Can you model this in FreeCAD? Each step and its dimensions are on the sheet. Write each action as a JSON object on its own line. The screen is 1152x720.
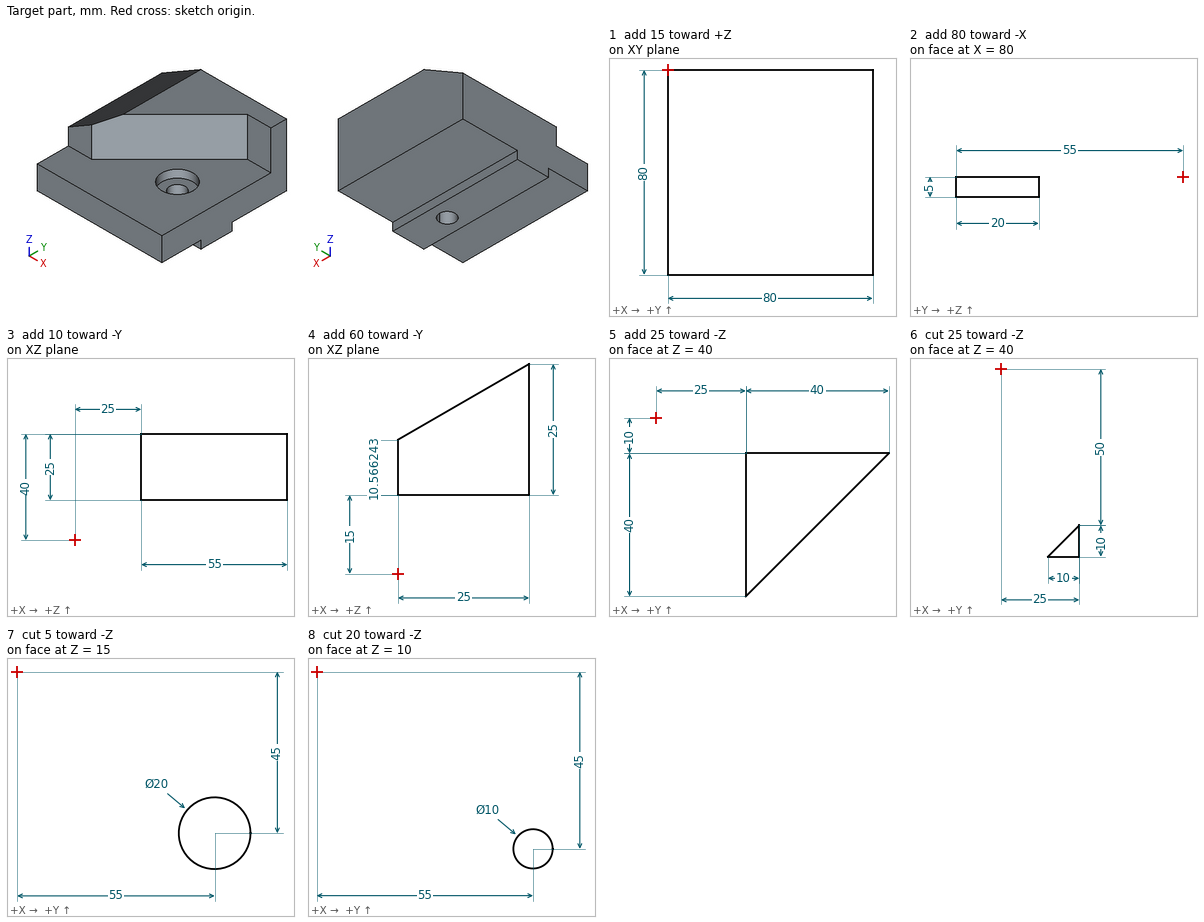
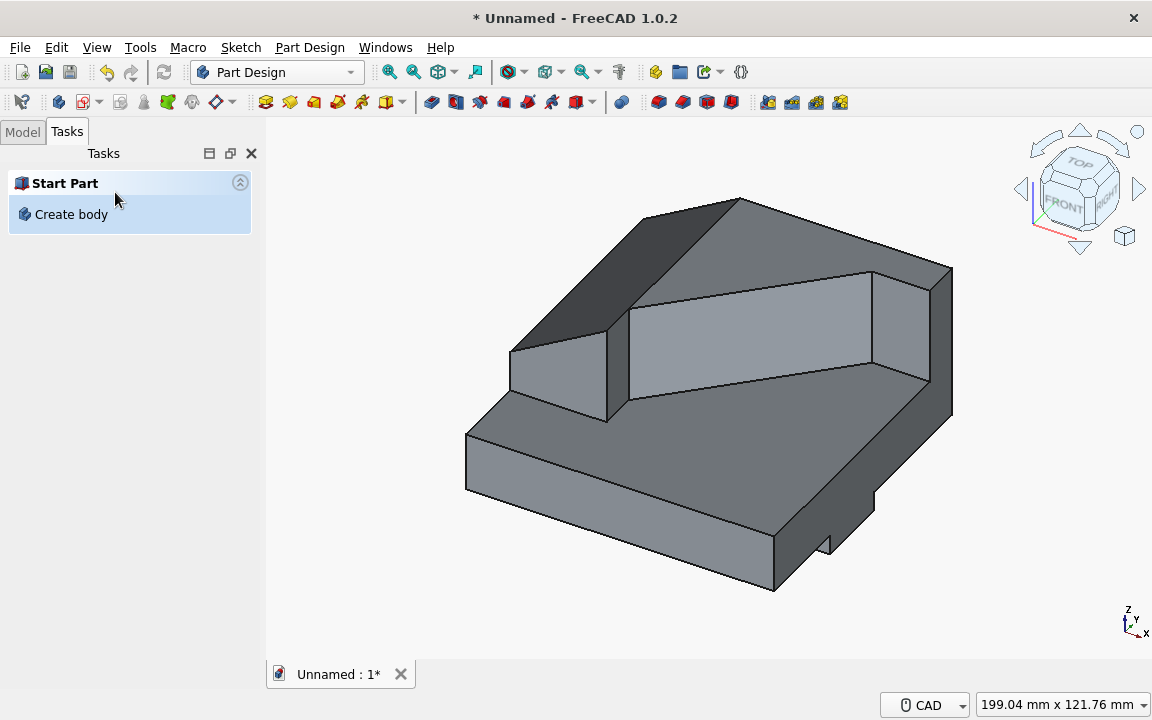
{"action": "left_click", "coordinate": [746, 252]}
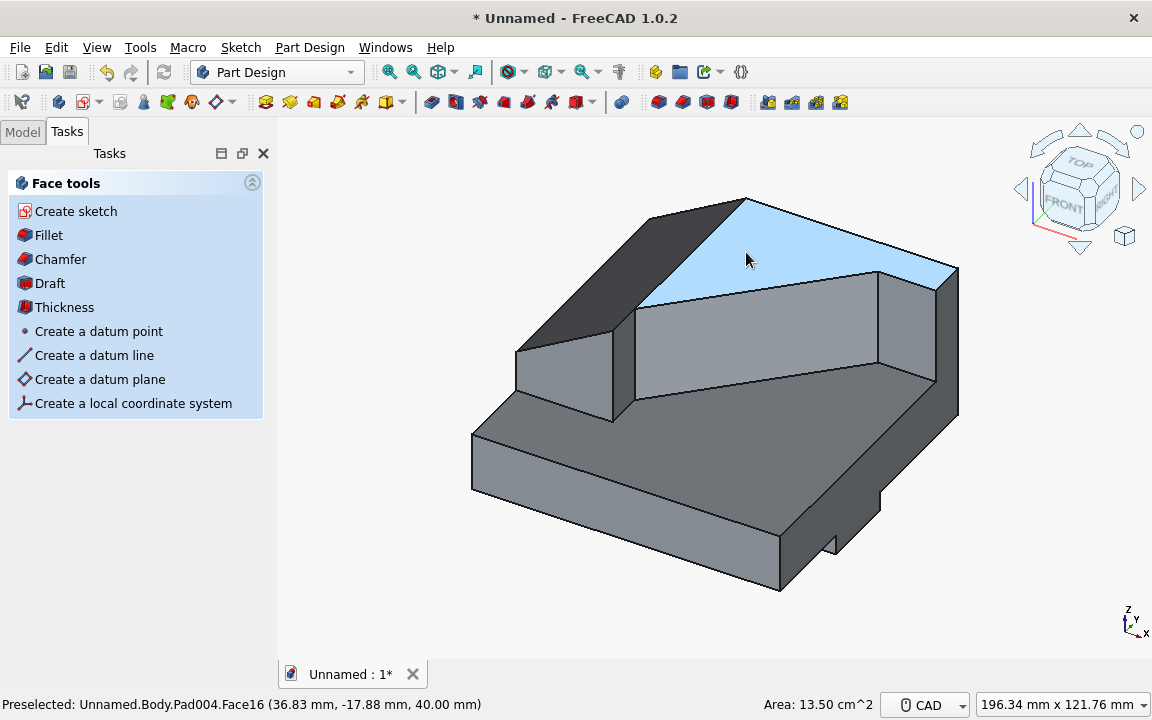
{"action": "left_click", "coordinate": [84, 102]}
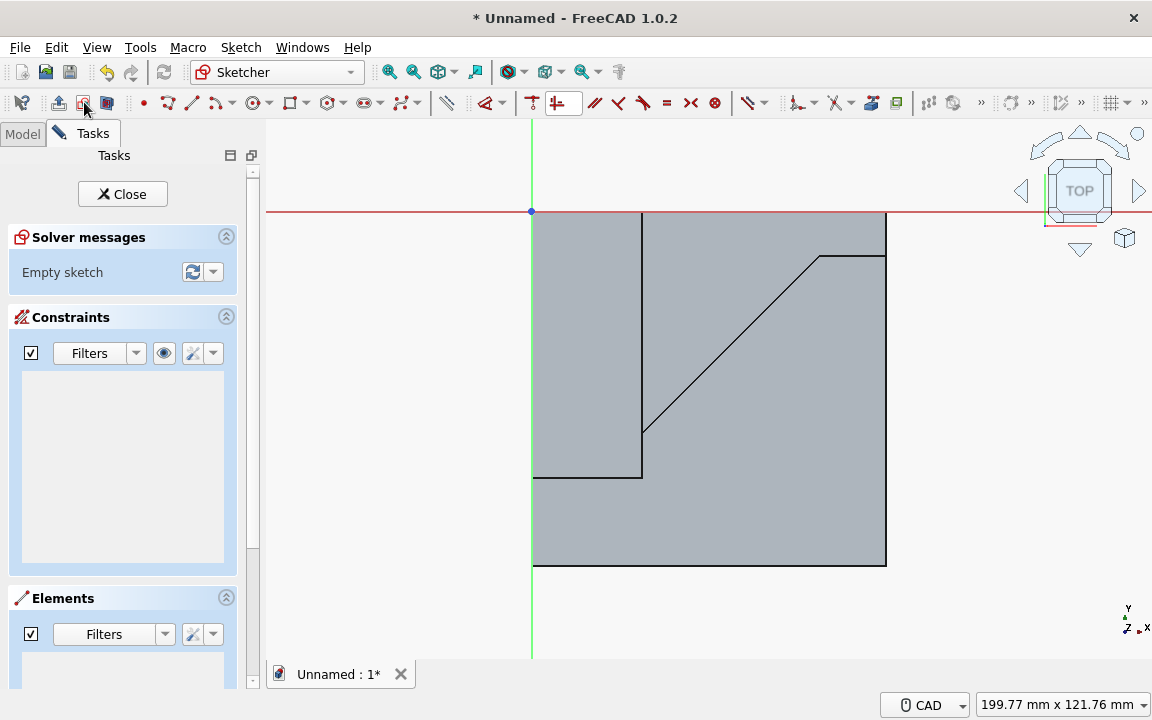
{"action": "scroll", "coordinate": [617, 466], "scroll_direction": "up", "scroll_amount": 10}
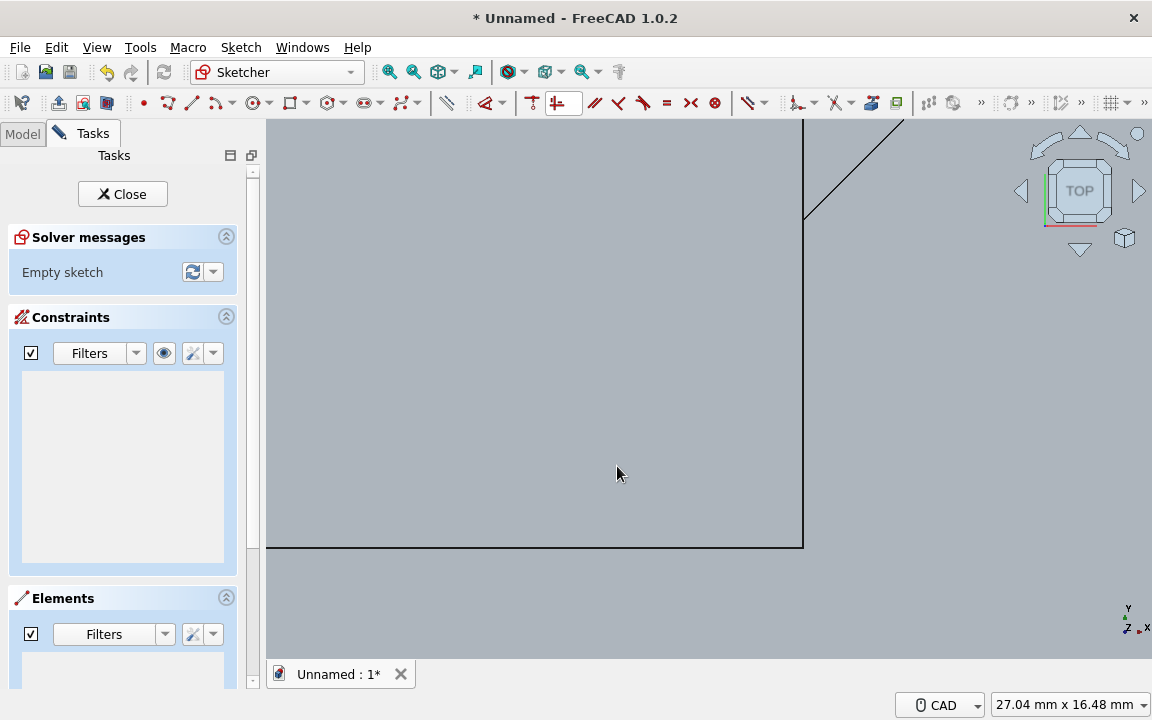
{"action": "left_click", "coordinate": [168, 104]}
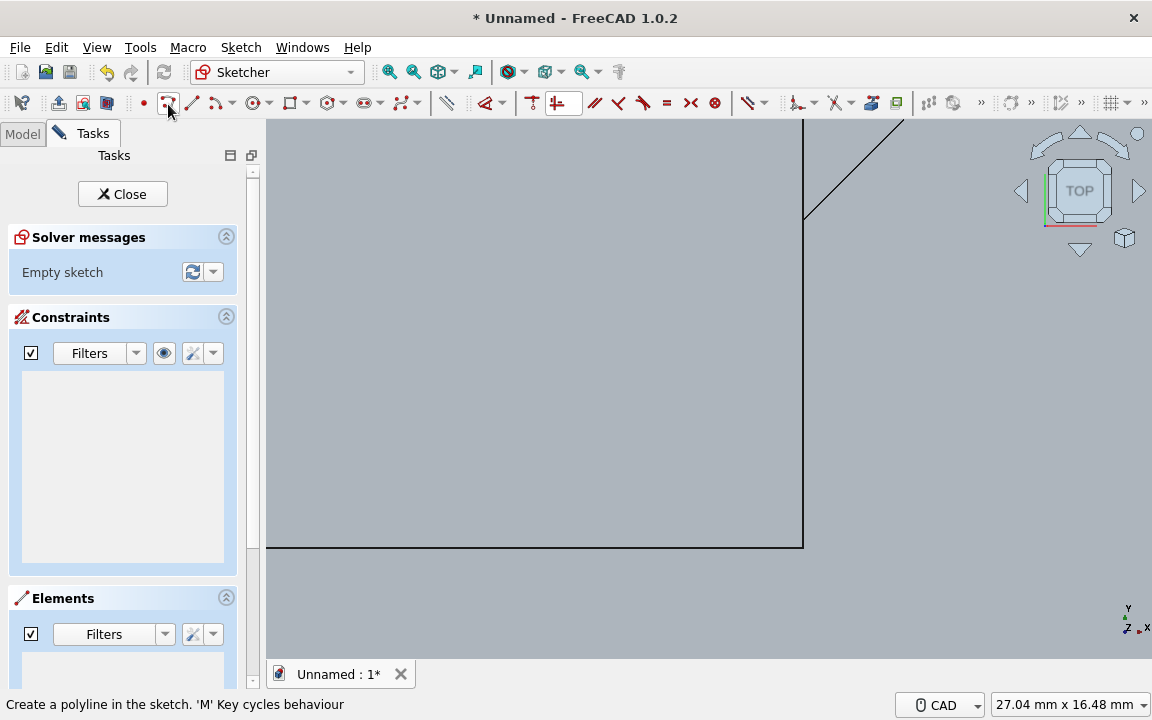
{"action": "left_click", "coordinate": [803, 221]}
{"action": "left_click", "coordinate": [475, 548]}
{"action": "left_click", "coordinate": [803, 548]}
{"action": "left_click", "coordinate": [803, 222]}
{"action": "key", "text": "Escape"}
{"action": "key", "text": "Escape"}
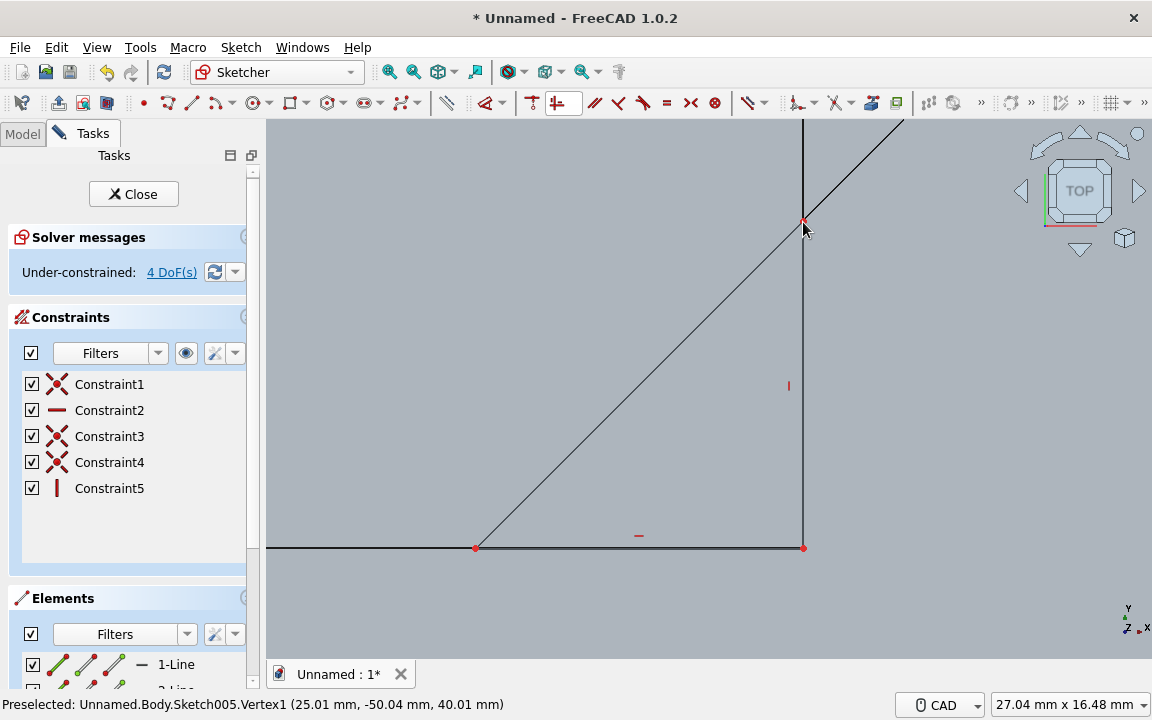
{"action": "left_click", "coordinate": [486, 104]}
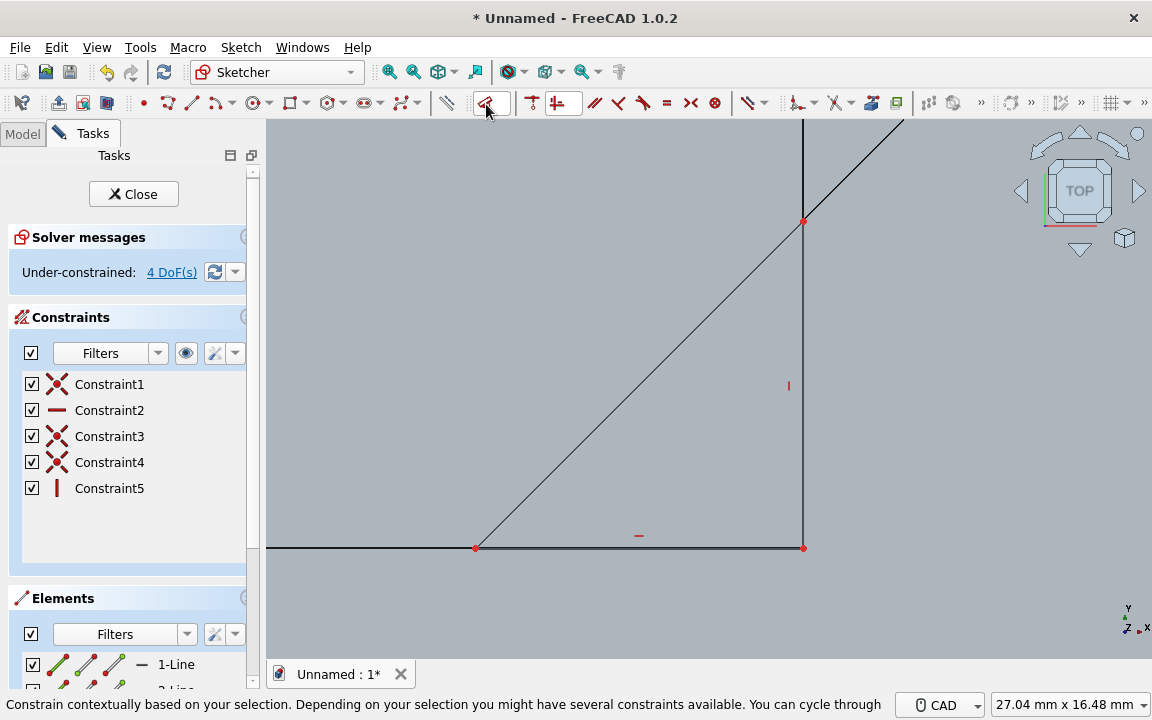
{"action": "left_click", "coordinate": [573, 549]}
{"action": "left_click", "coordinate": [639, 583]}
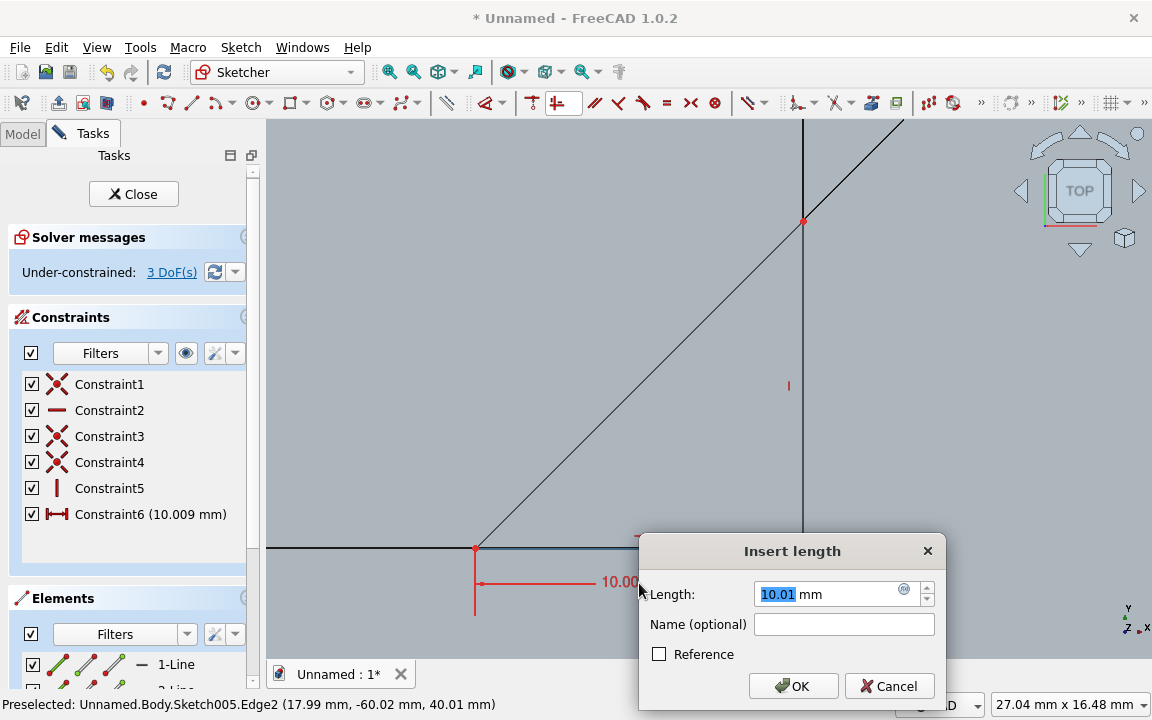
{"action": "type", "text": "10"}
{"action": "key", "text": "Return"}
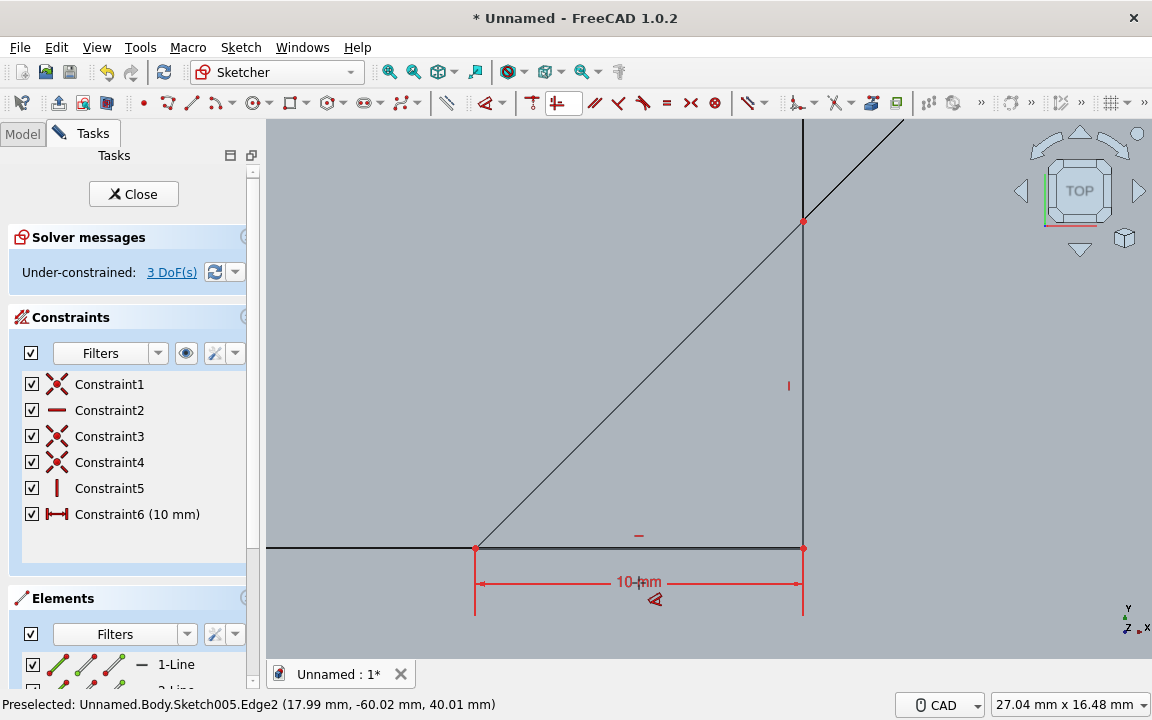
{"action": "left_click", "coordinate": [803, 451]}
{"action": "left_click", "coordinate": [837, 386]}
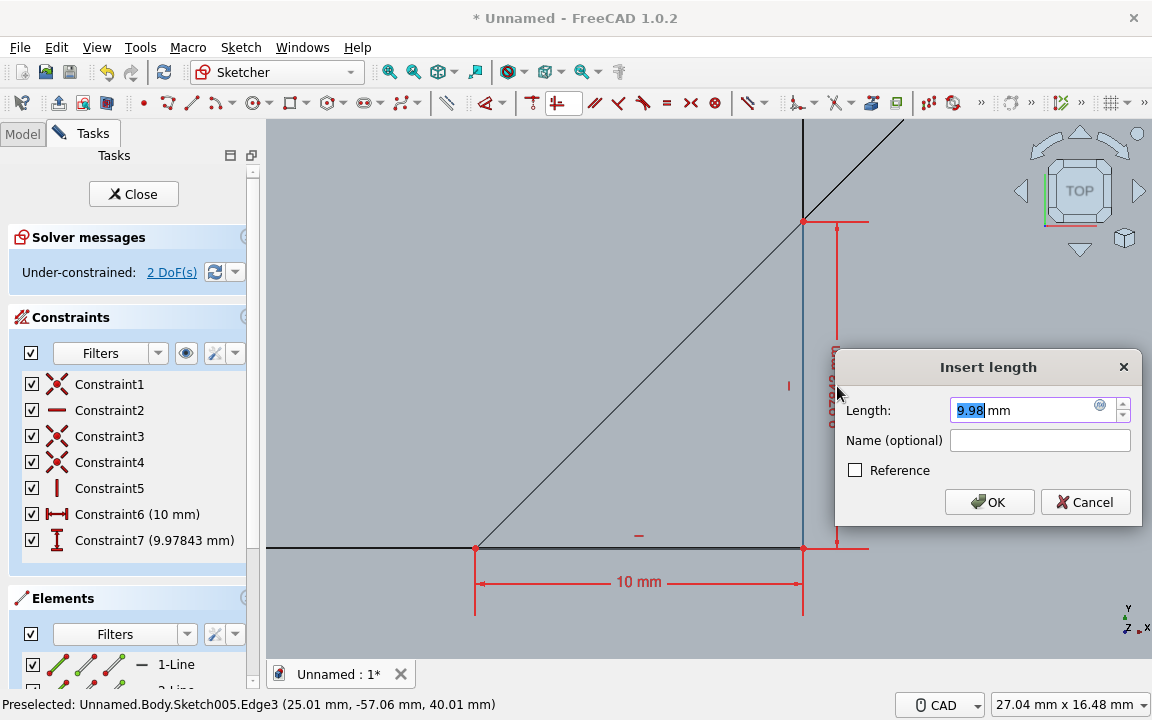
{"action": "type", "text": "10"}
{"action": "key", "text": "Return"}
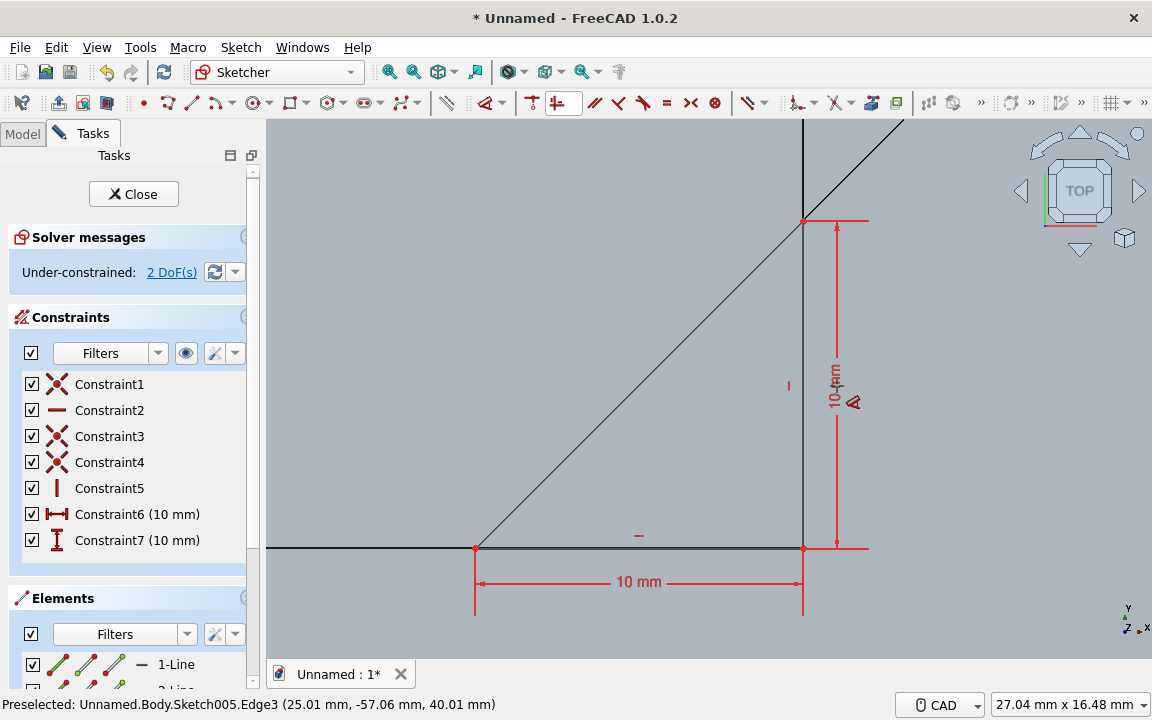
{"action": "left_click", "coordinate": [803, 221]}
{"action": "left_click", "coordinate": [549, 255]}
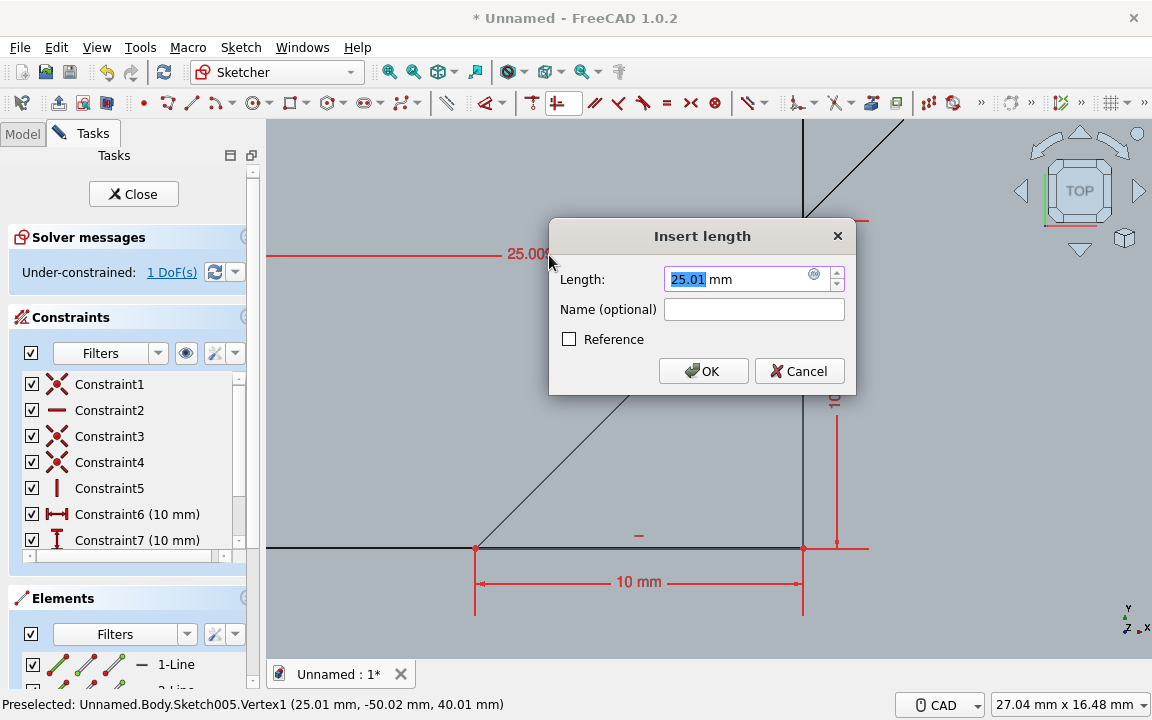
{"action": "type", "text": "25"}
{"action": "key", "text": "Return"}